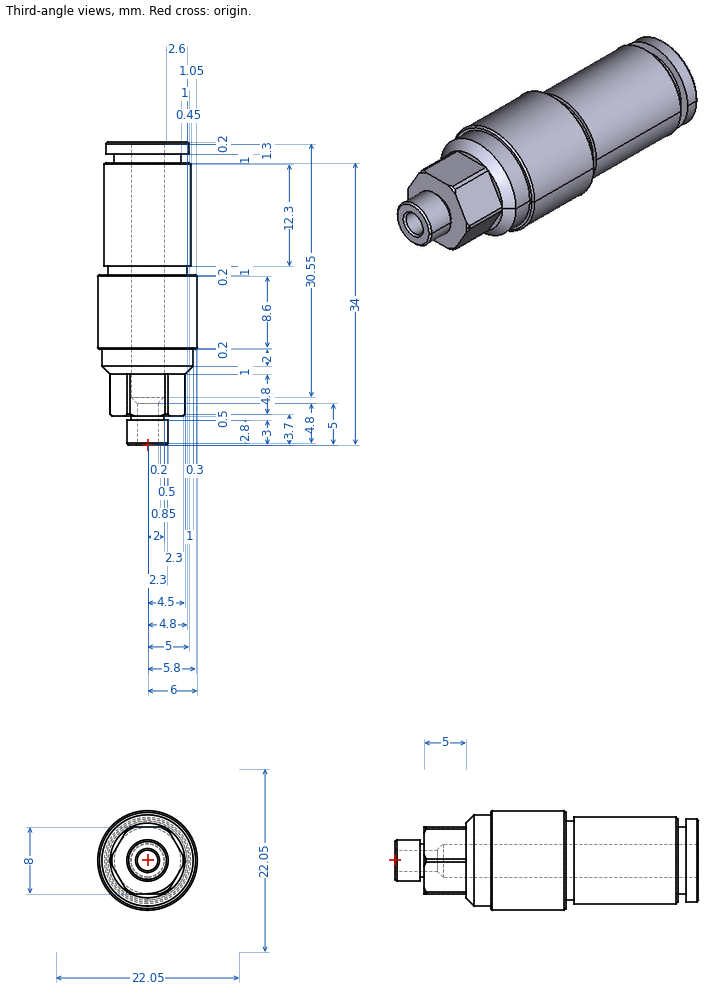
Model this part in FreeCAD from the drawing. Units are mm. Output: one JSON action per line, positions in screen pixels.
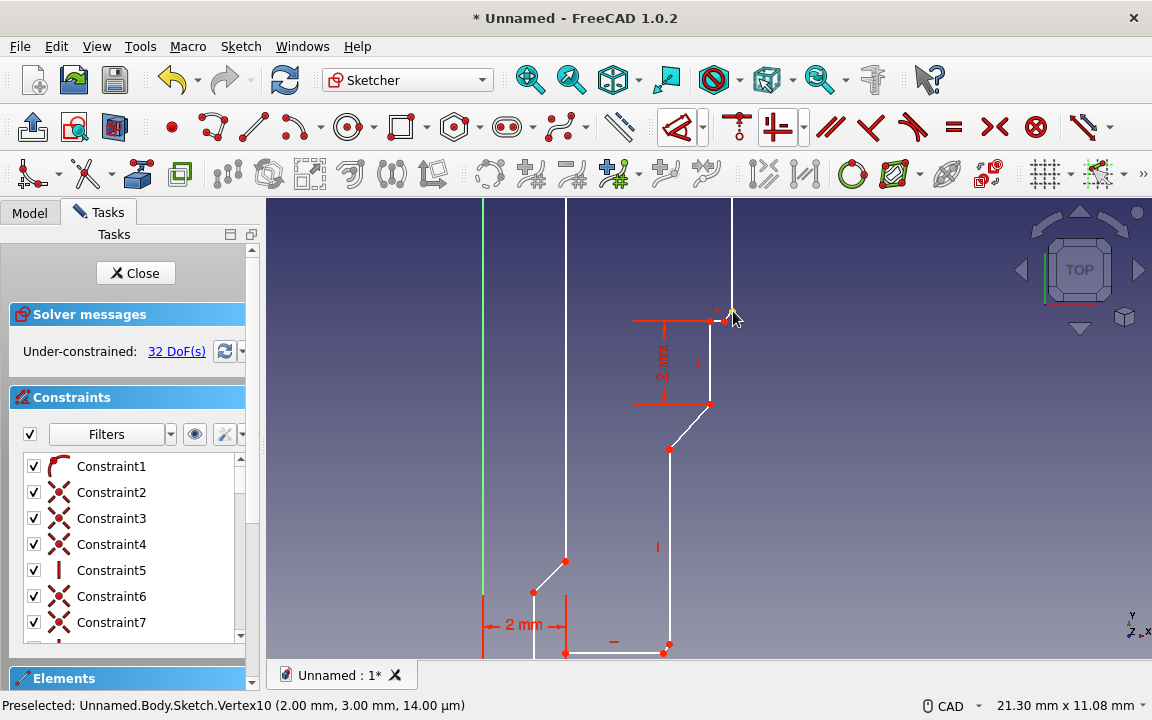
{"action": "left_click", "coordinate": [732, 311]}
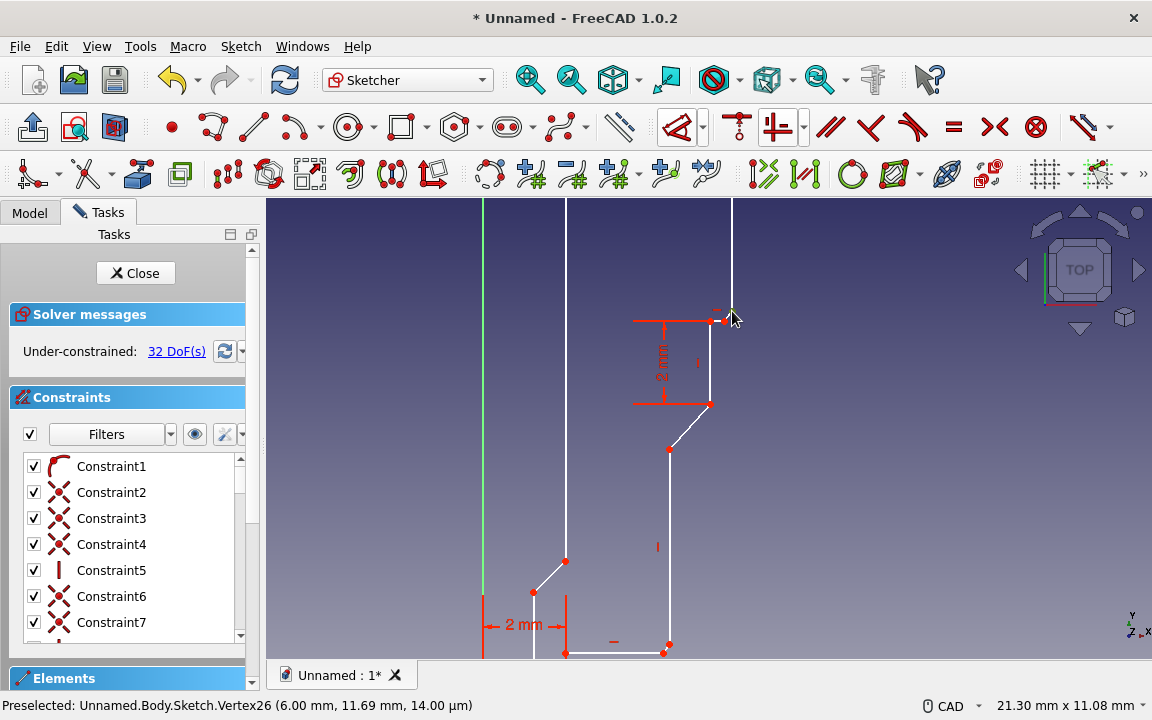
{"action": "key", "text": "l"}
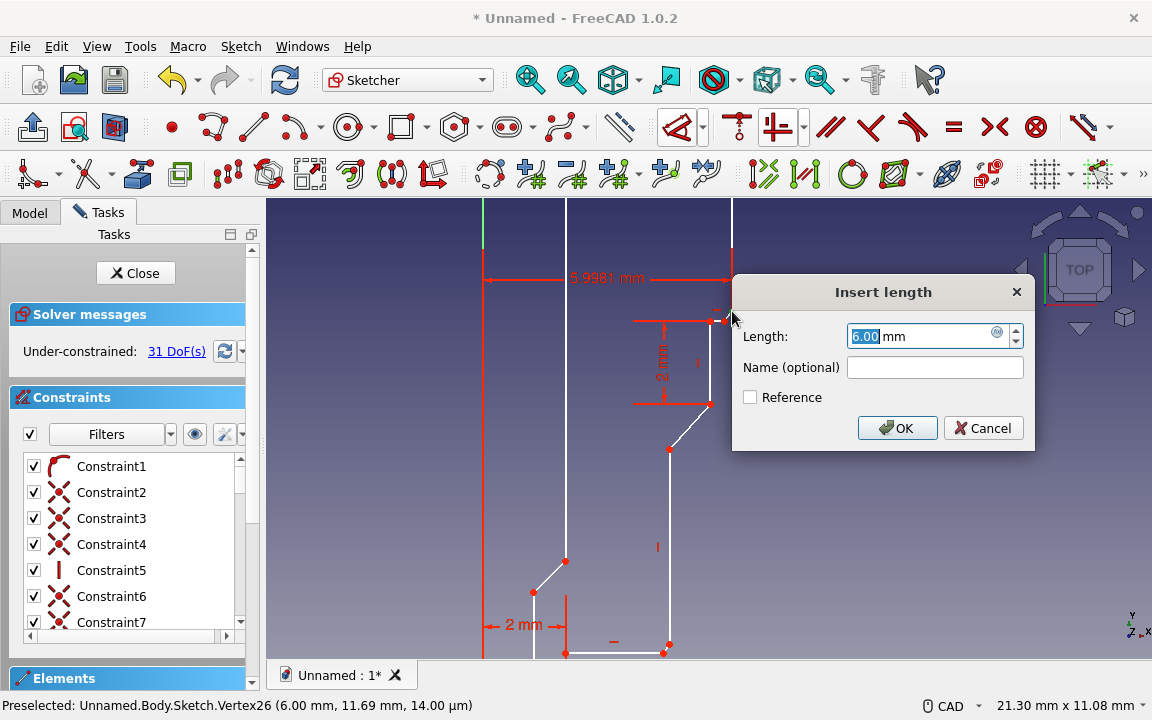
{"action": "type", "text": "6"}
{"action": "key", "text": "Return"}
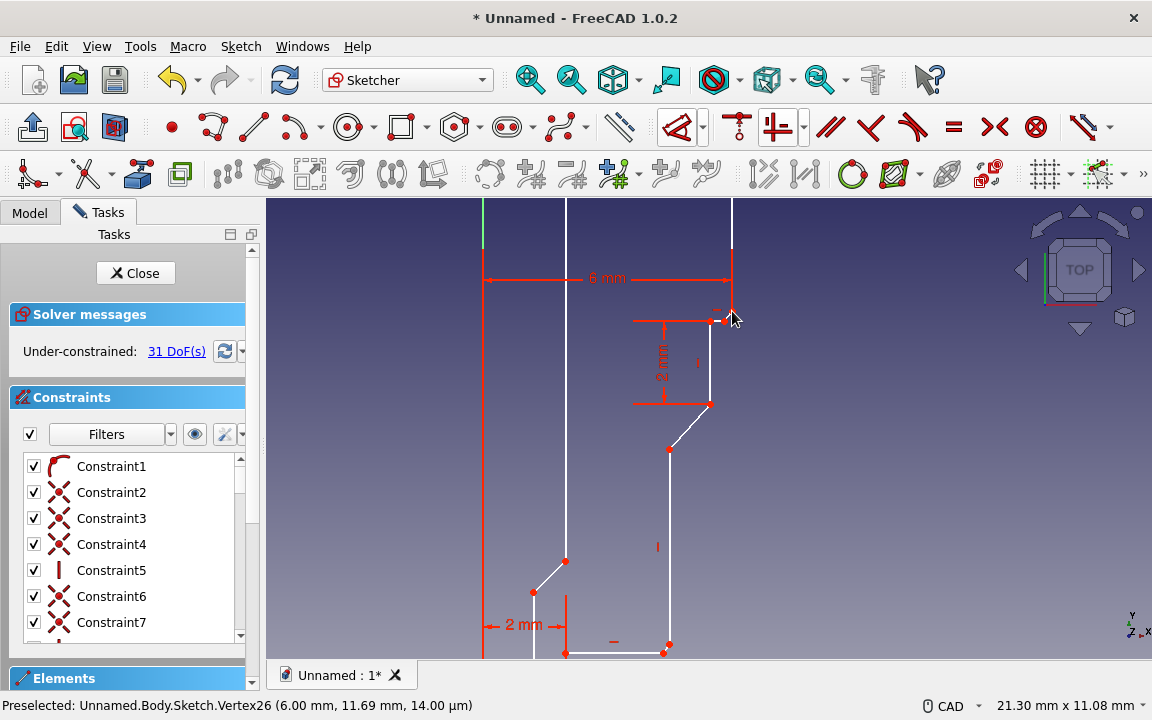
{"action": "scroll", "coordinate": [649, 527], "scroll_direction": "down", "scroll_amount": 8}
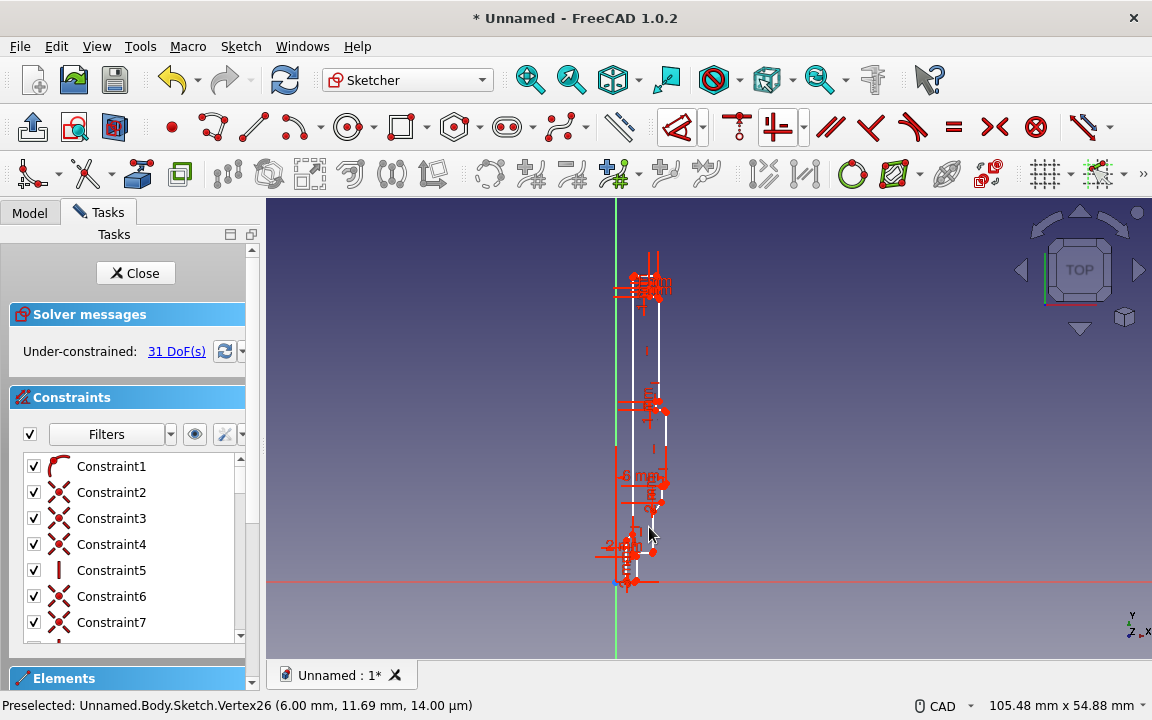
{"action": "scroll", "coordinate": [658, 297], "scroll_direction": "up", "scroll_amount": 7}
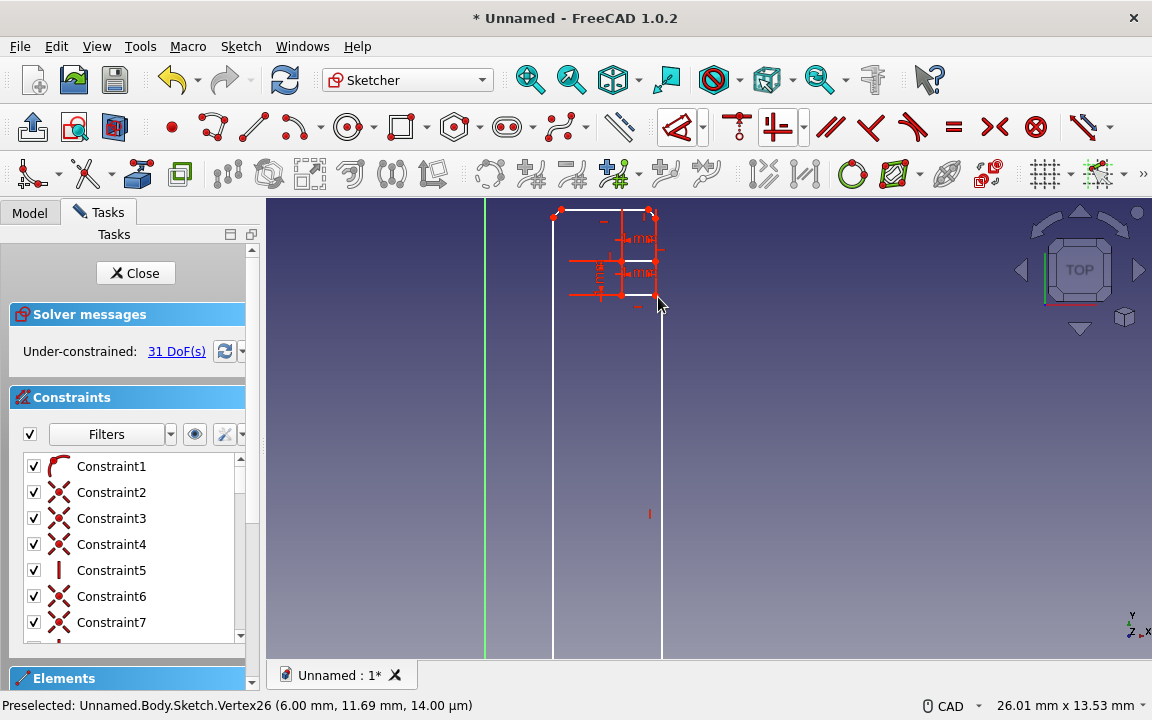
{"action": "left_click", "coordinate": [656, 295]}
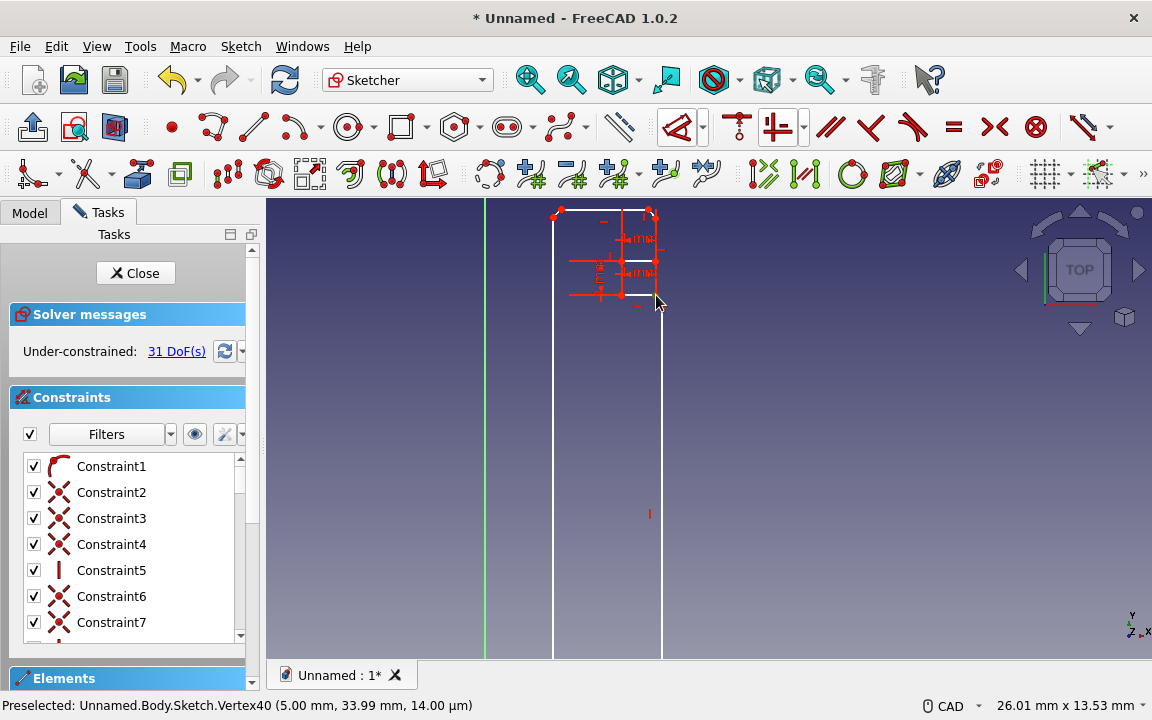
{"action": "key", "text": "l"}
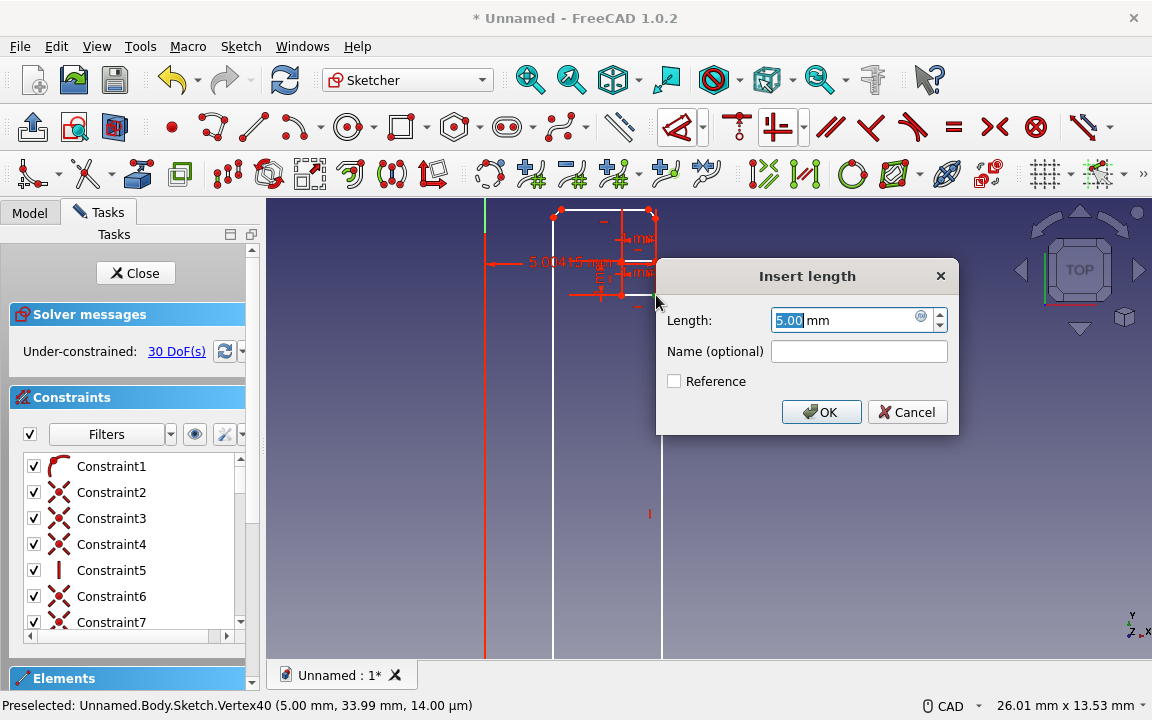
{"action": "type", "text": "5"}
{"action": "key", "text": "Return"}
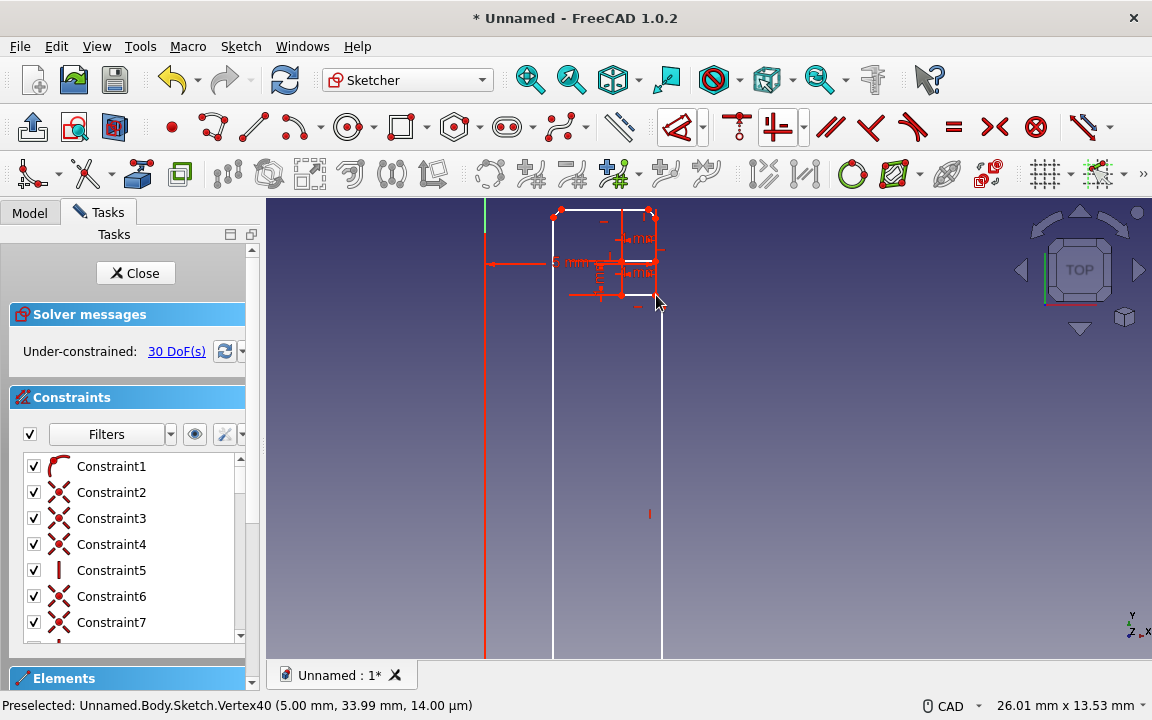
{"action": "scroll", "coordinate": [658, 297], "scroll_direction": "down", "scroll_amount": 7}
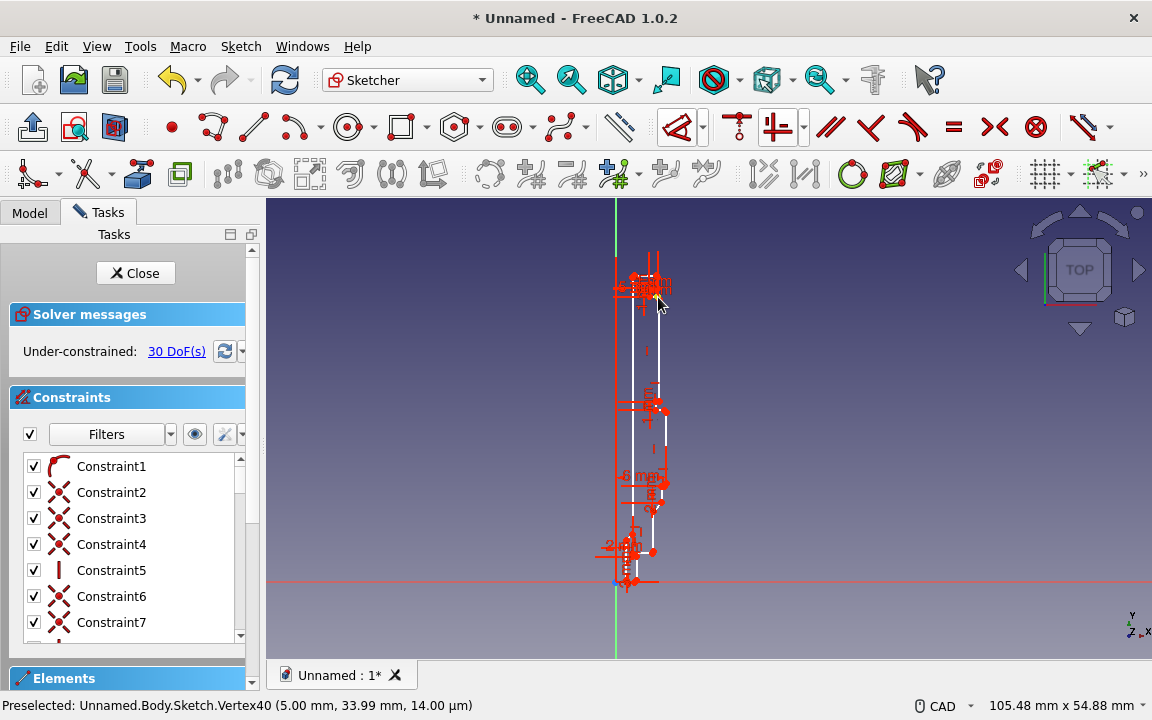
{"action": "scroll", "coordinate": [633, 277], "scroll_direction": "up", "scroll_amount": 8}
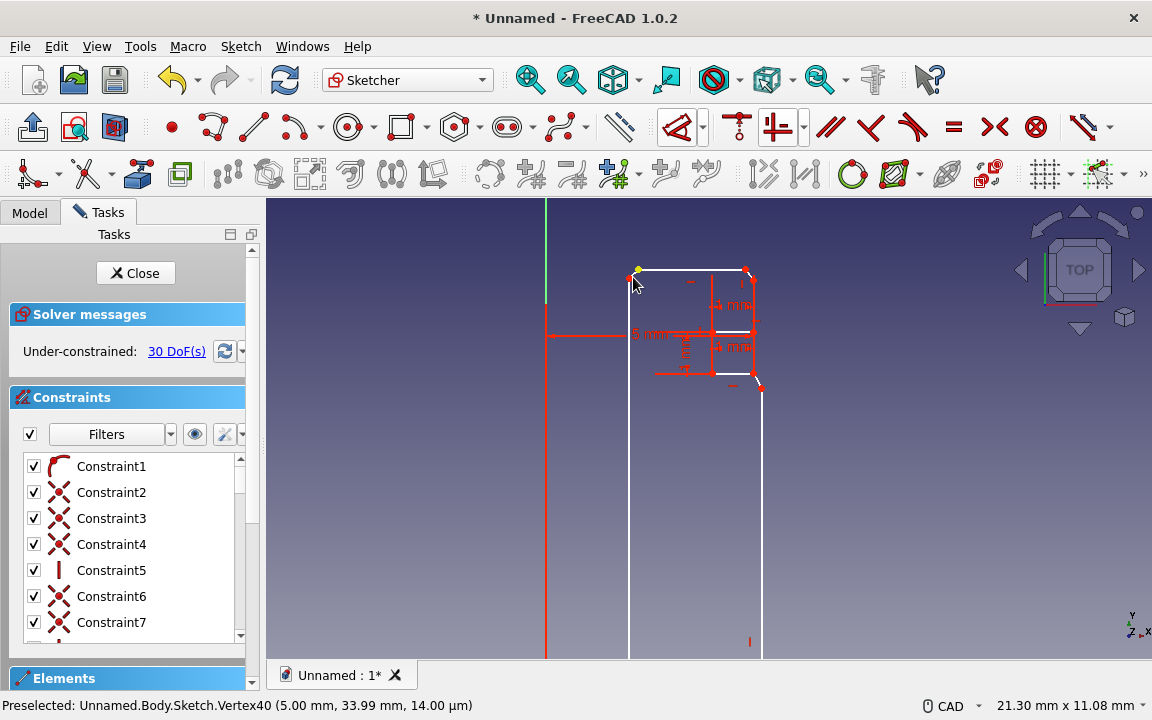
{"action": "left_click", "coordinate": [629, 279]}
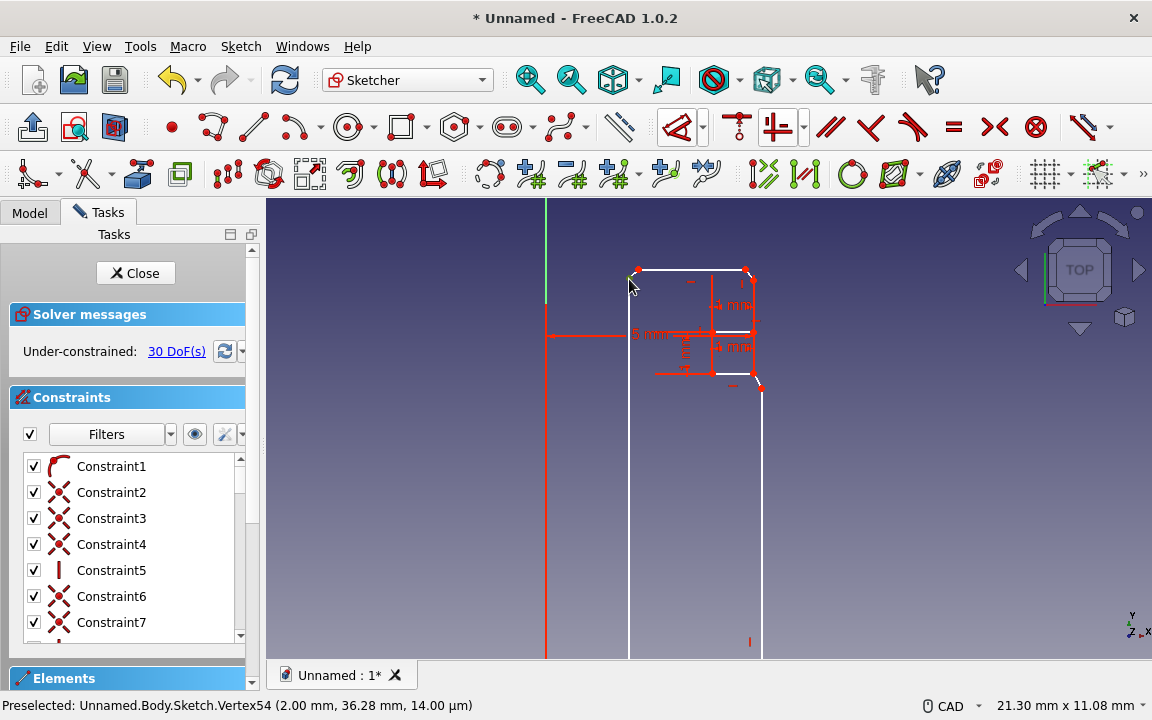
{"action": "left_click", "coordinate": [702, 128]}